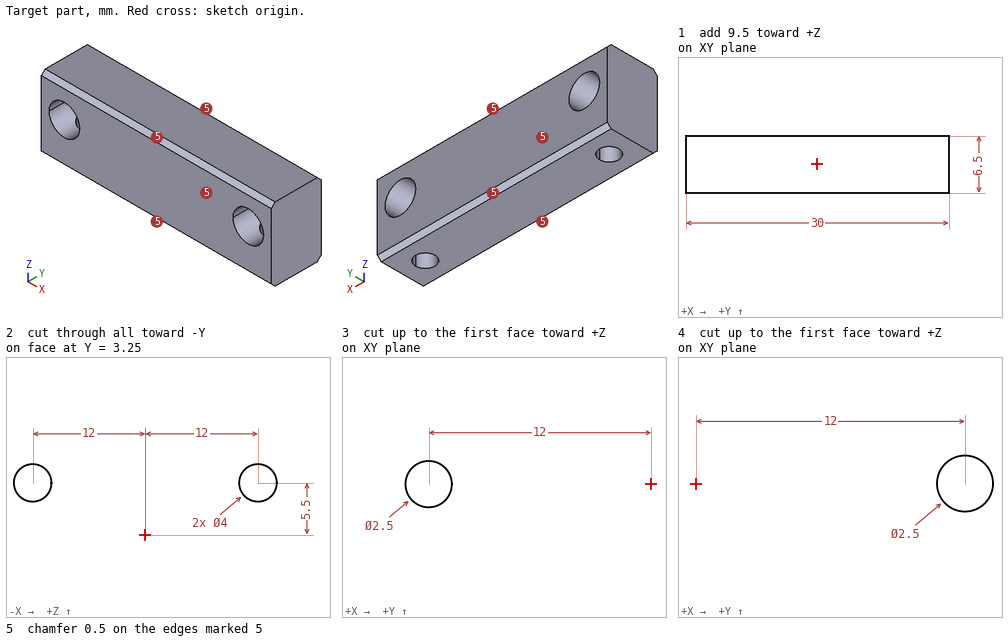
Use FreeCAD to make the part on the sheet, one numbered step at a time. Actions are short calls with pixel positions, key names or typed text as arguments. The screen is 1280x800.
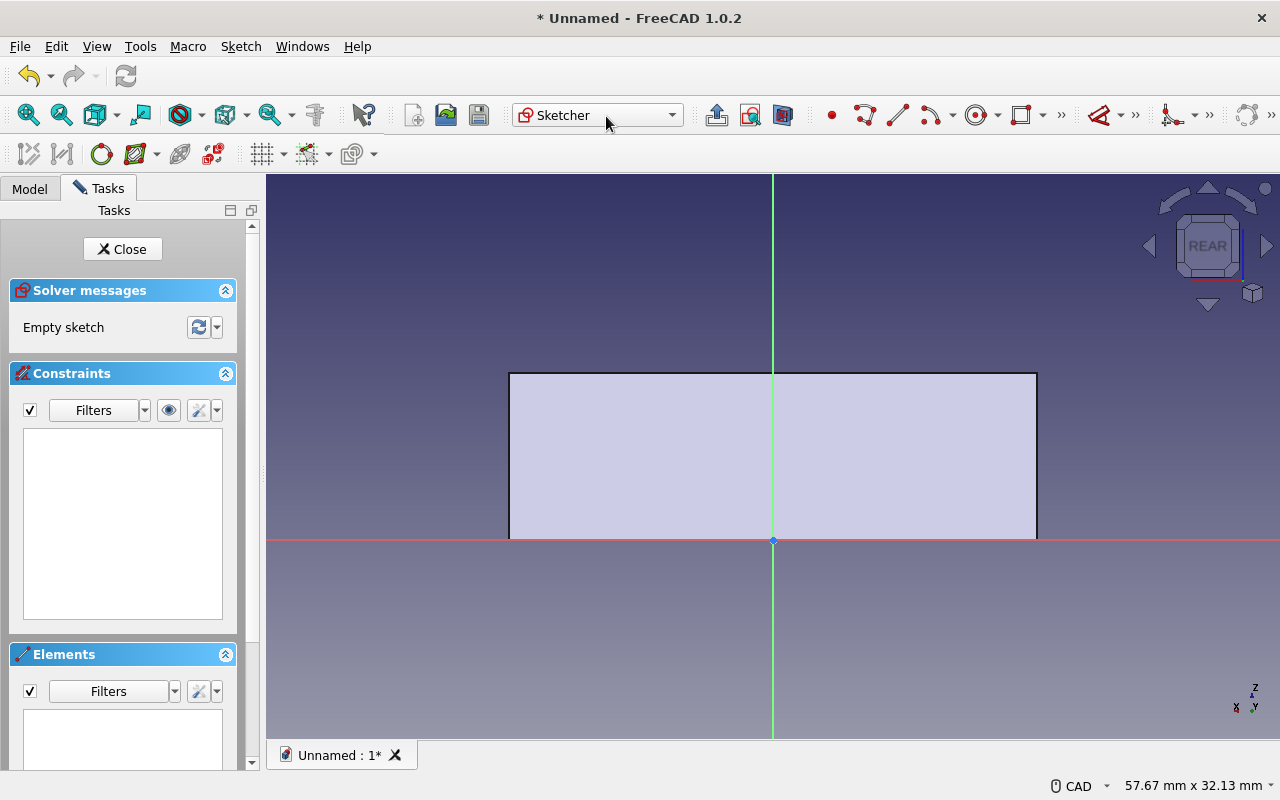
key(g)
key(c)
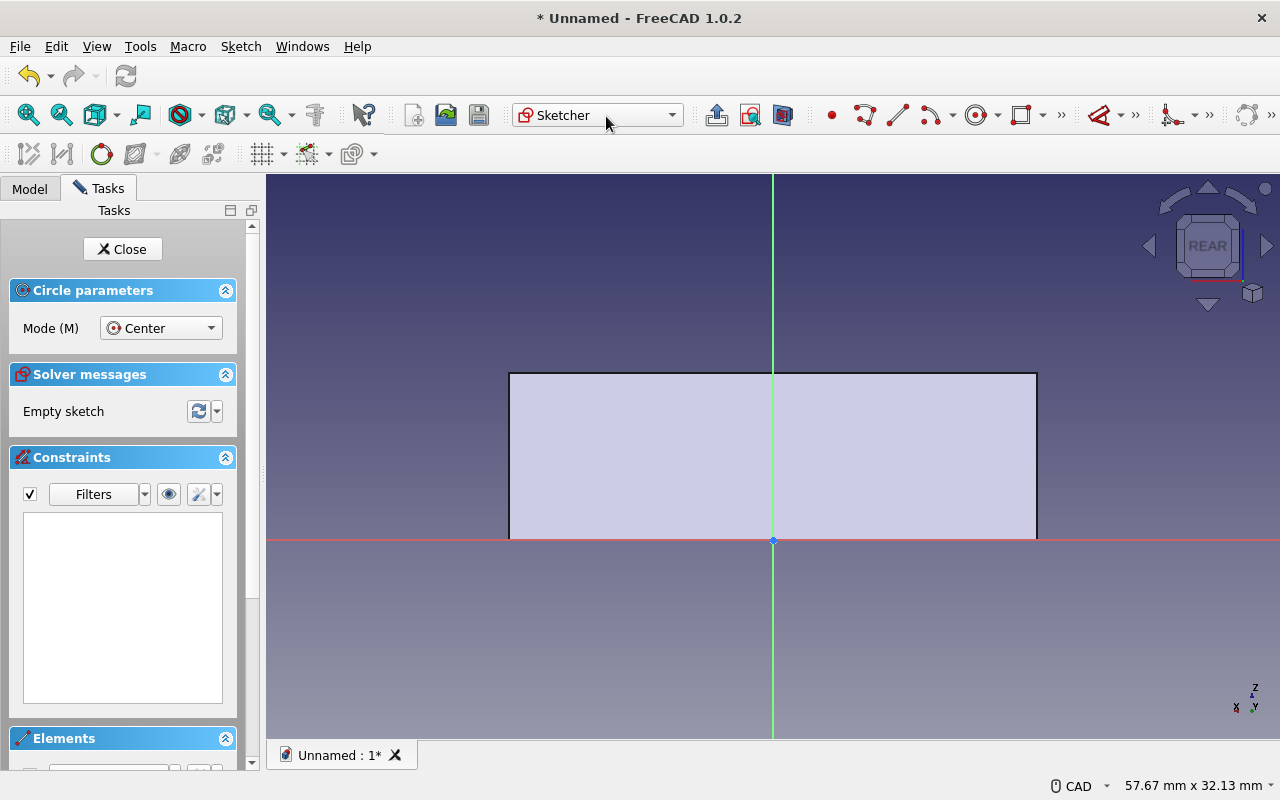
click(984, 443)
click(1009, 418)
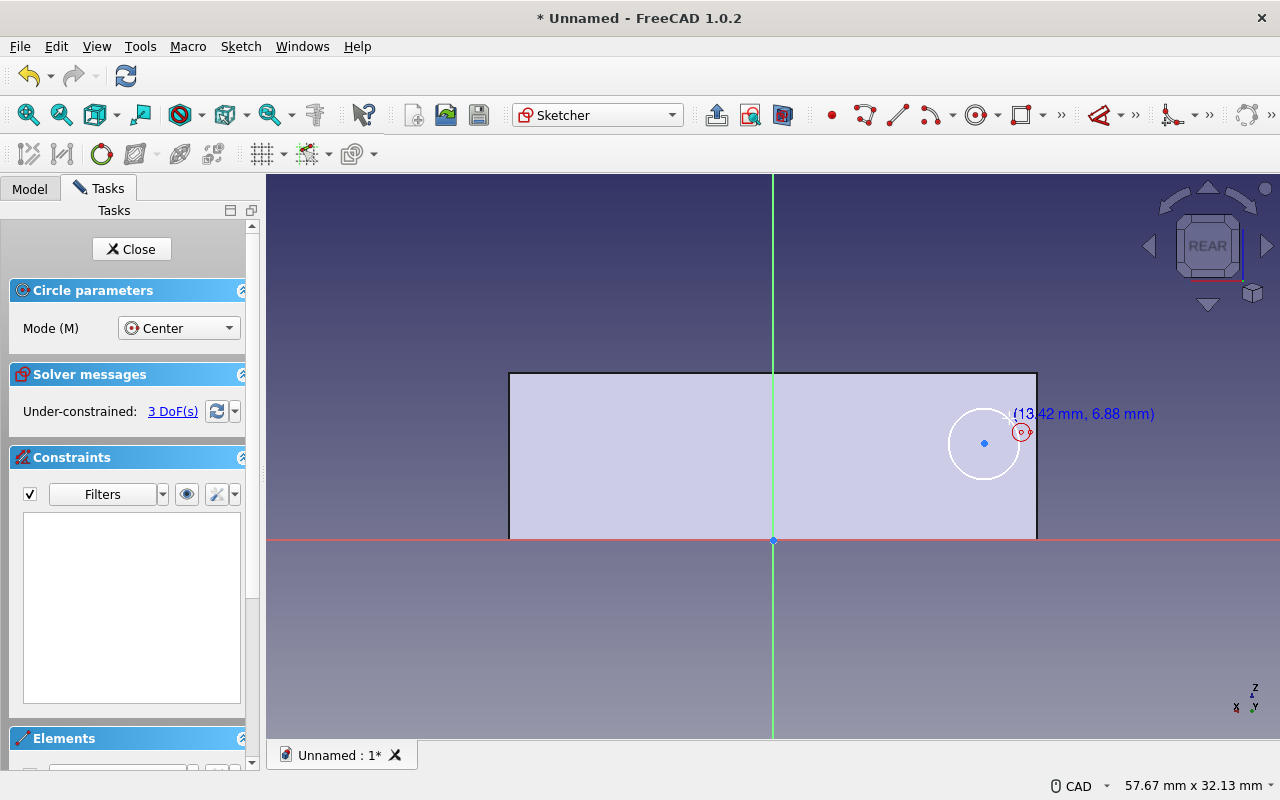
click(562, 443)
click(587, 418)
key(Escape)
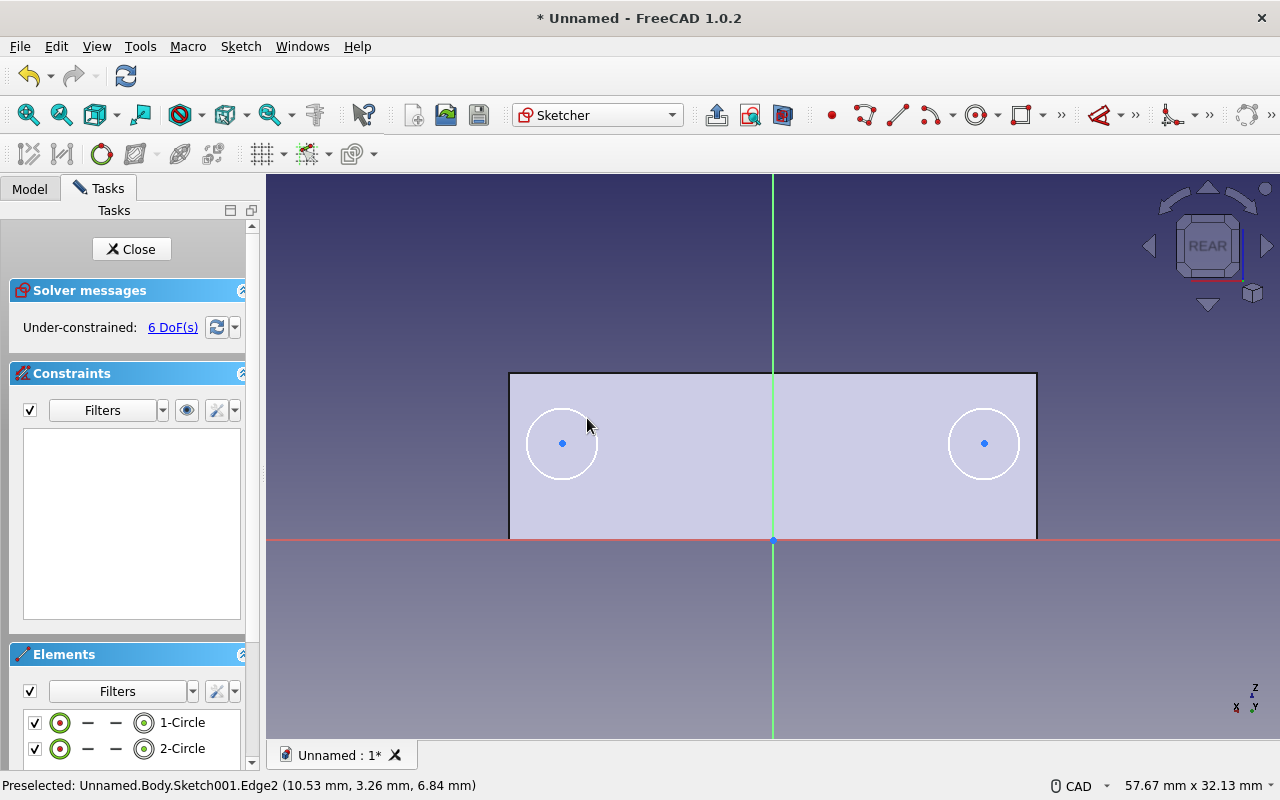
click(1009, 419)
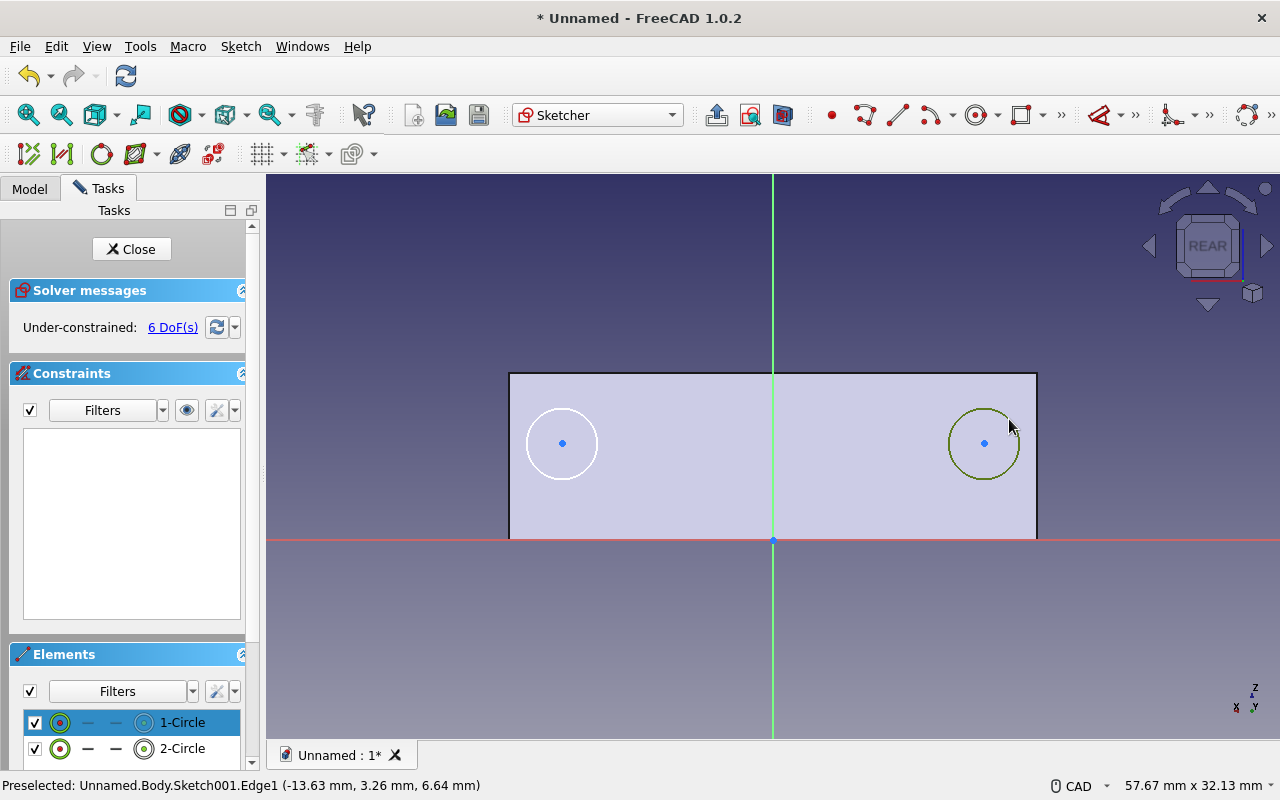
click(587, 419)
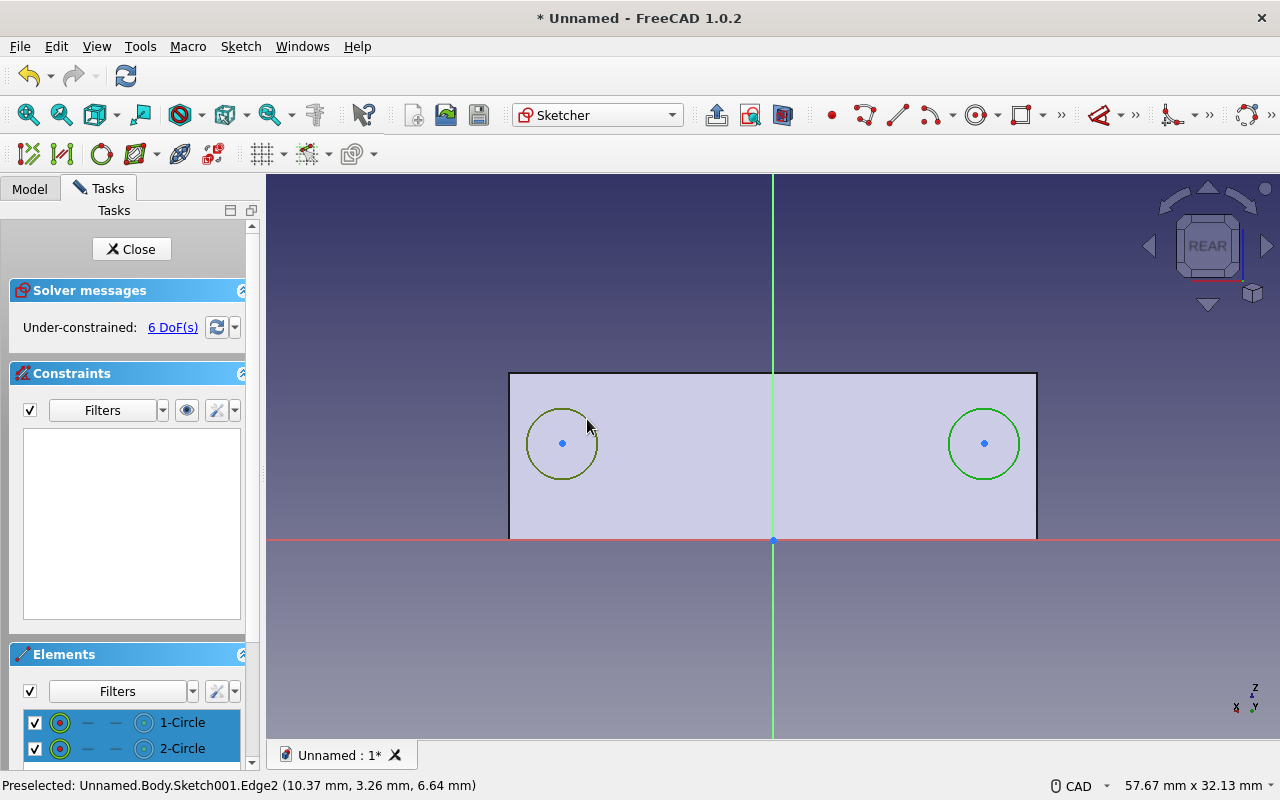
key(e)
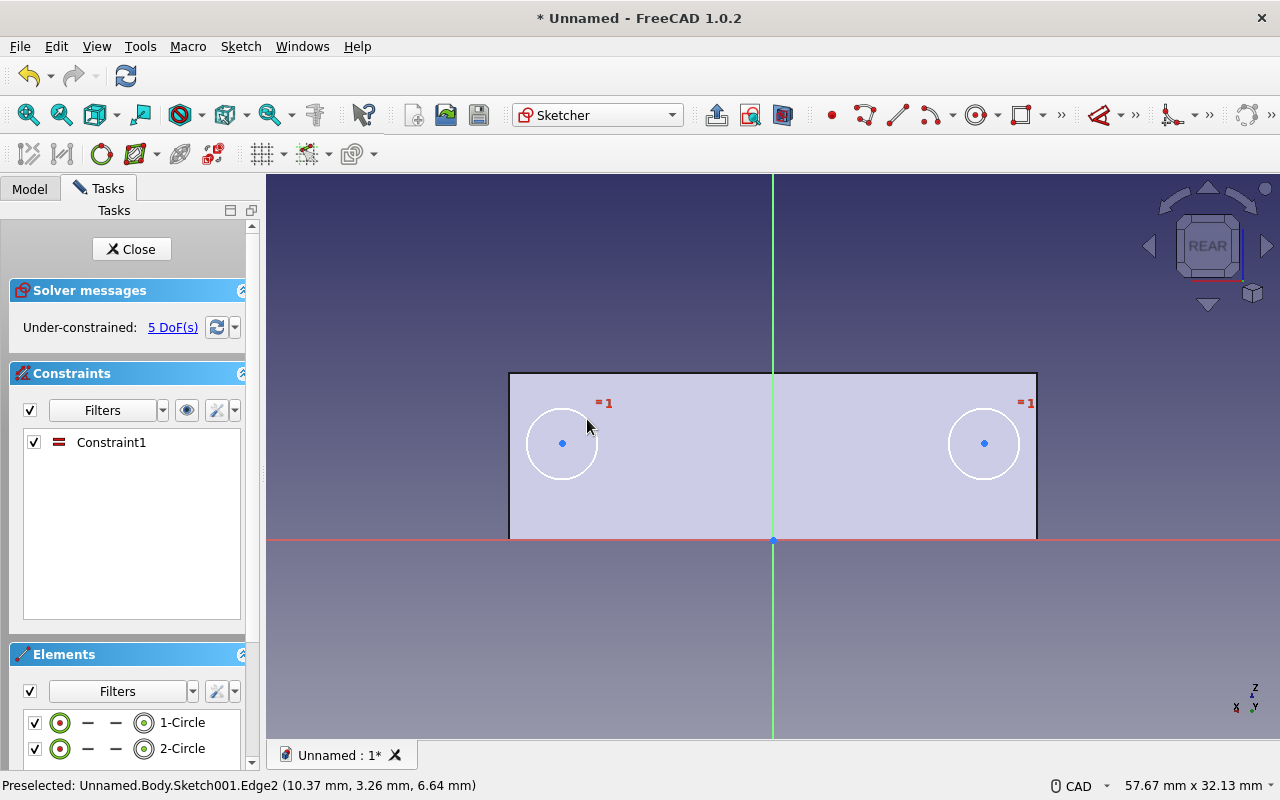
click(984, 444)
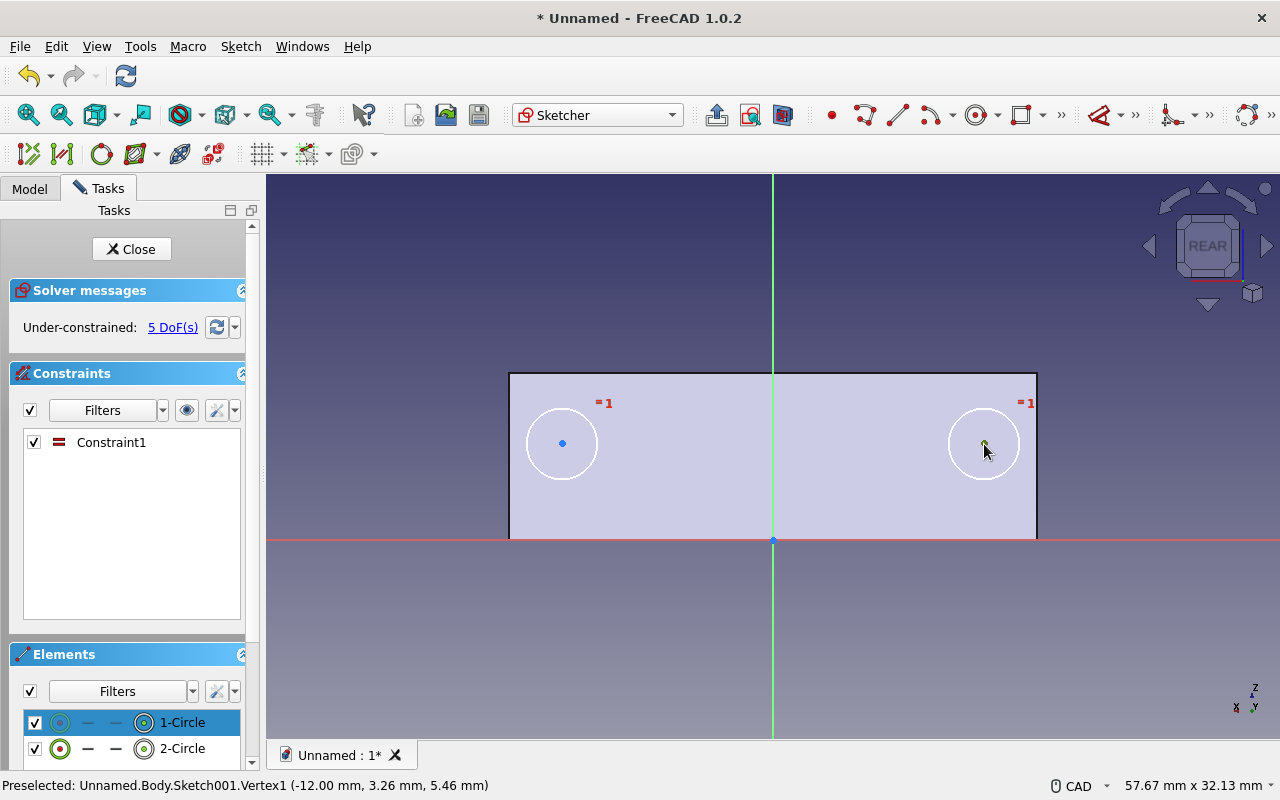
click(562, 444)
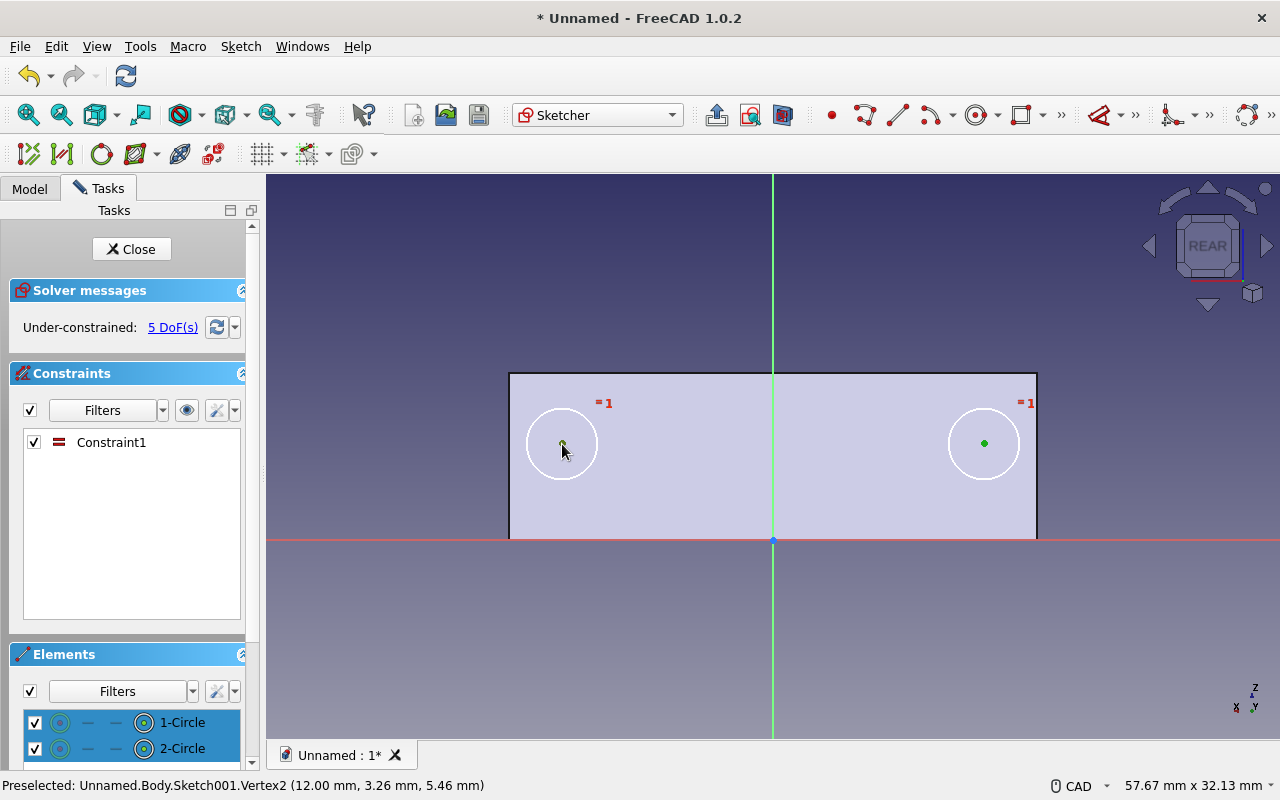
key(h)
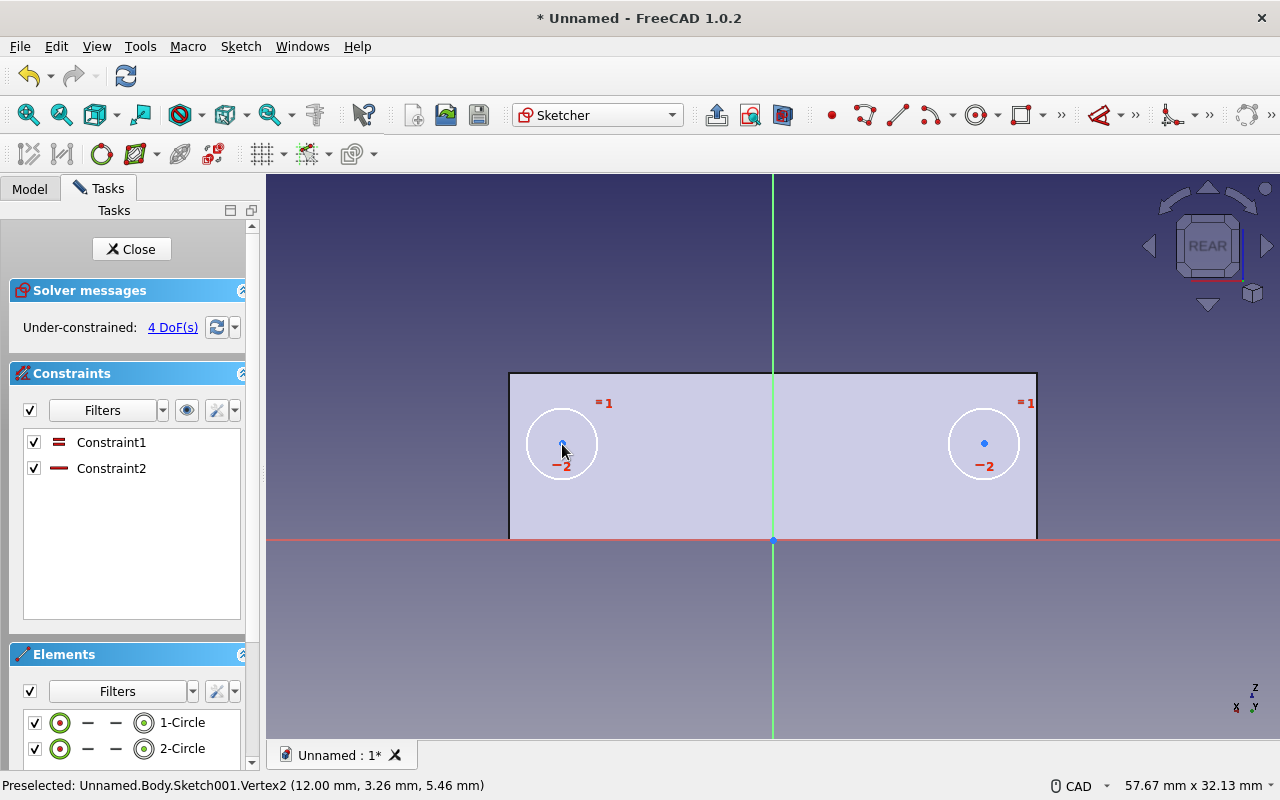
key(d)